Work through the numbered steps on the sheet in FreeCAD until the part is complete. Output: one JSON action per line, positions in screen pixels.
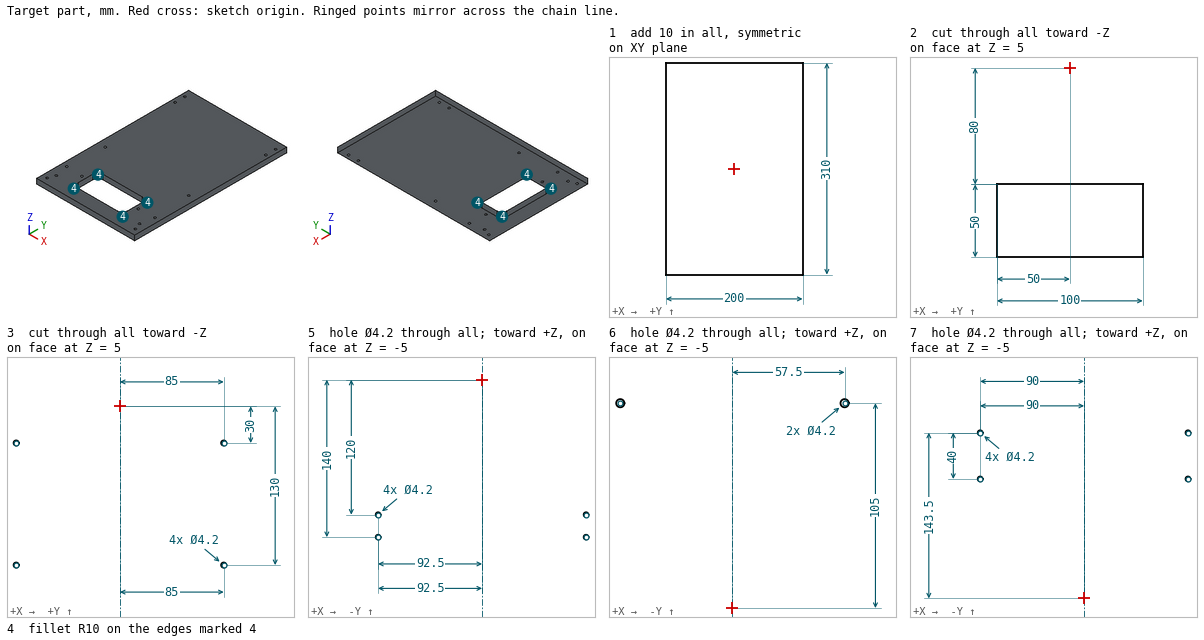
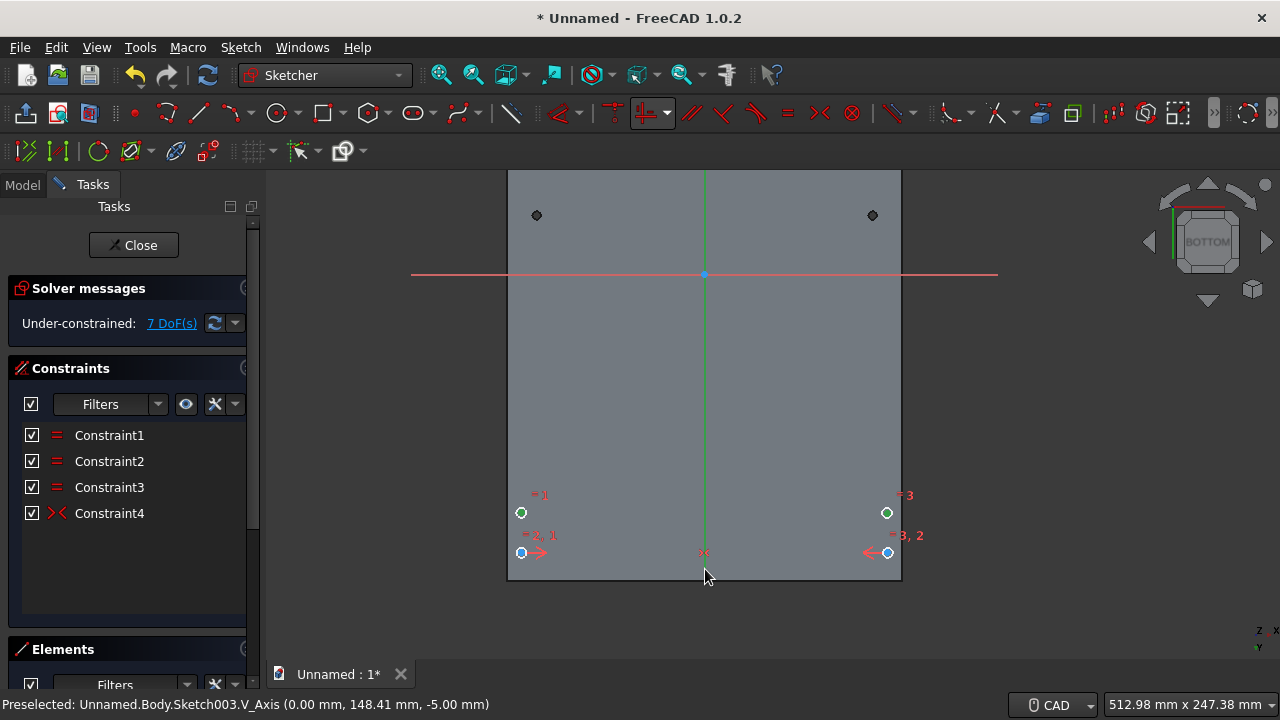
{"action": "left_click", "coordinate": [820, 114]}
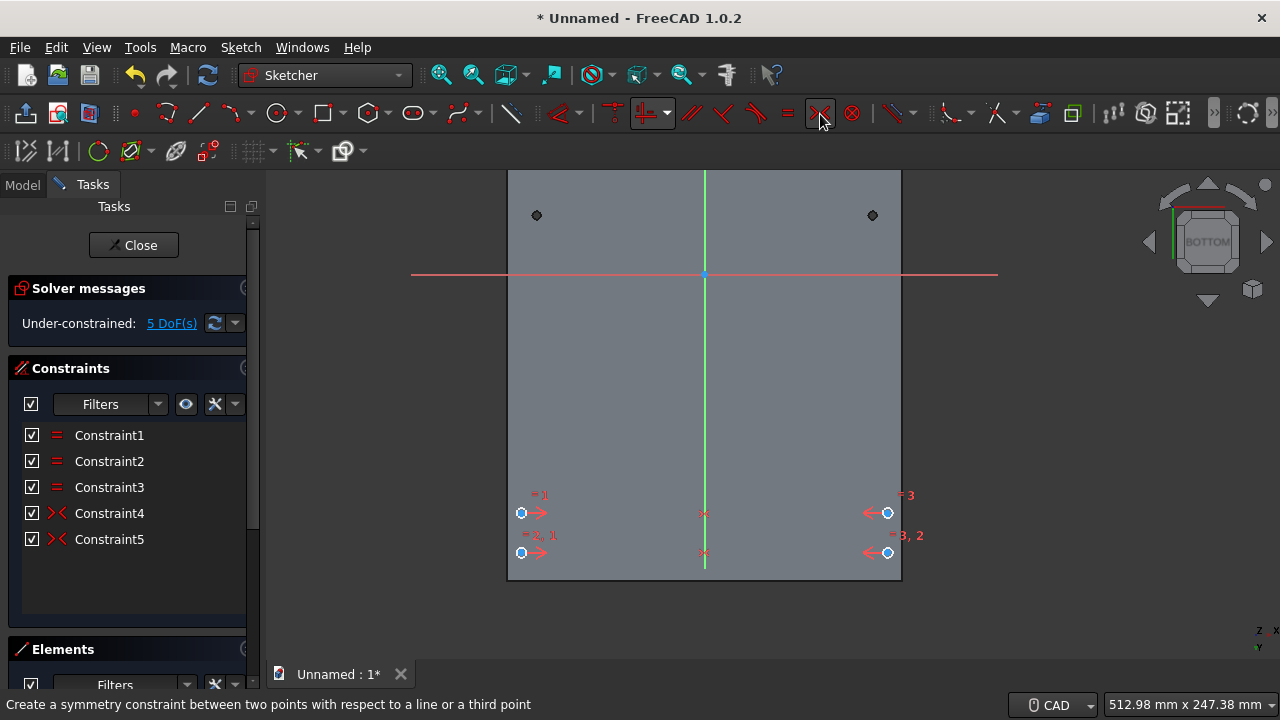
{"action": "left_click", "coordinate": [558, 114]}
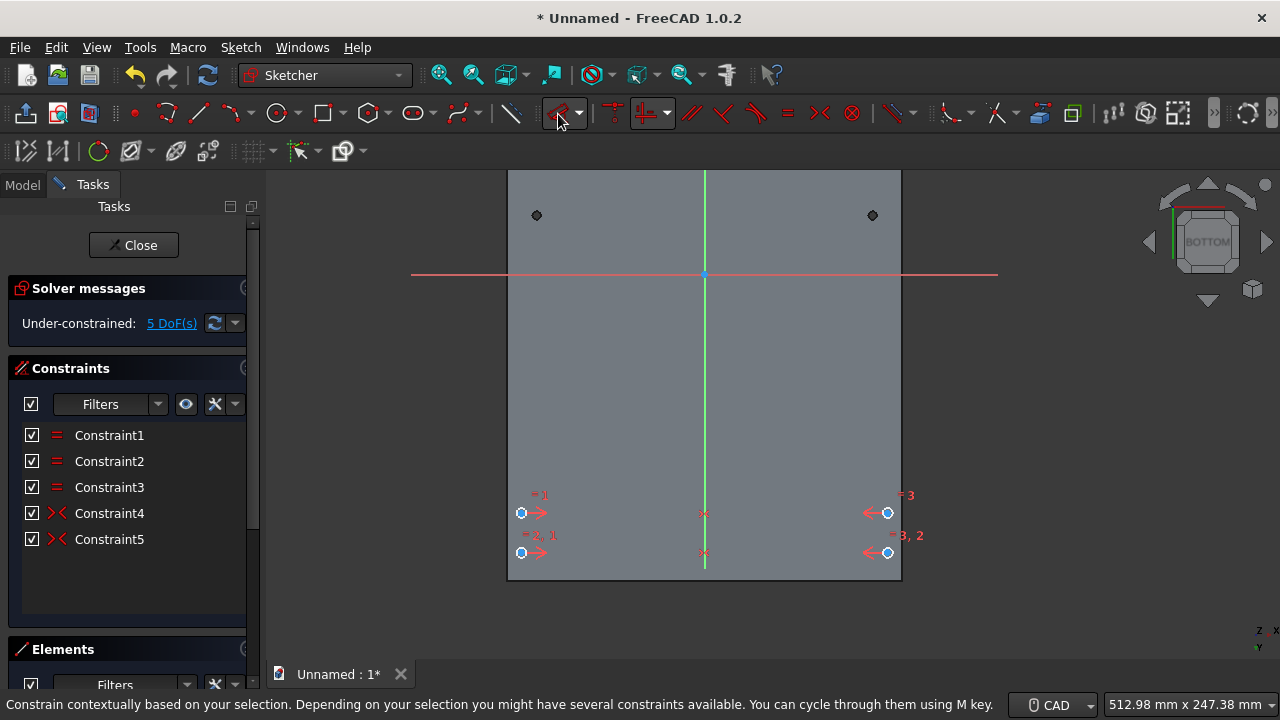
{"action": "scroll", "coordinate": [525, 510], "scroll_direction": "up", "scroll_amount": 8}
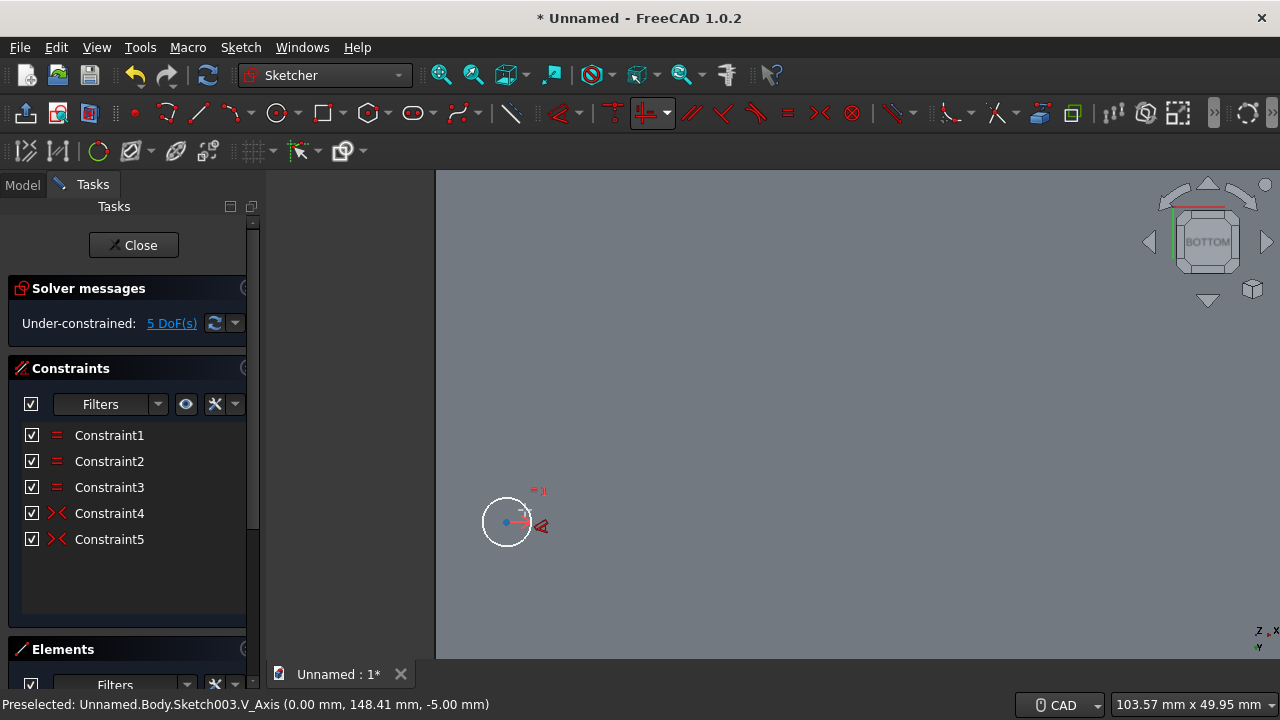
{"action": "left_click", "coordinate": [524, 505]}
{"action": "left_click", "coordinate": [547, 482]}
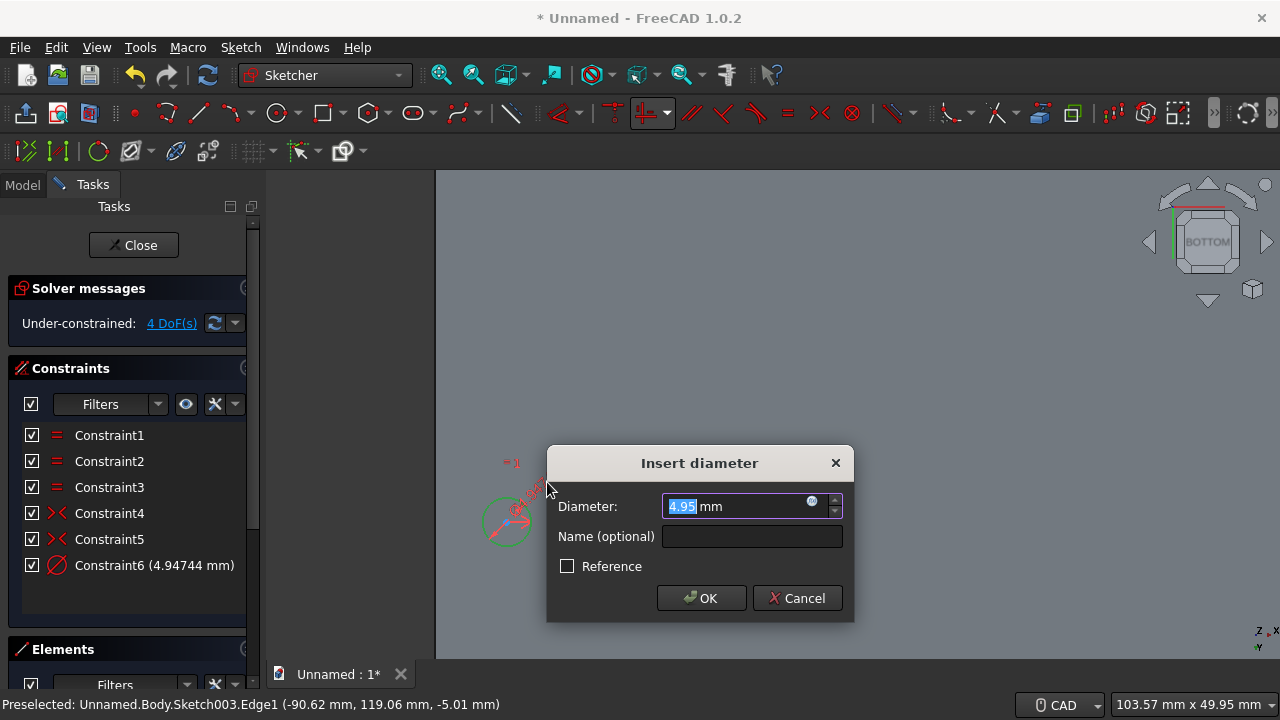
{"action": "type", "text": "4.2"}
{"action": "key", "text": "Return"}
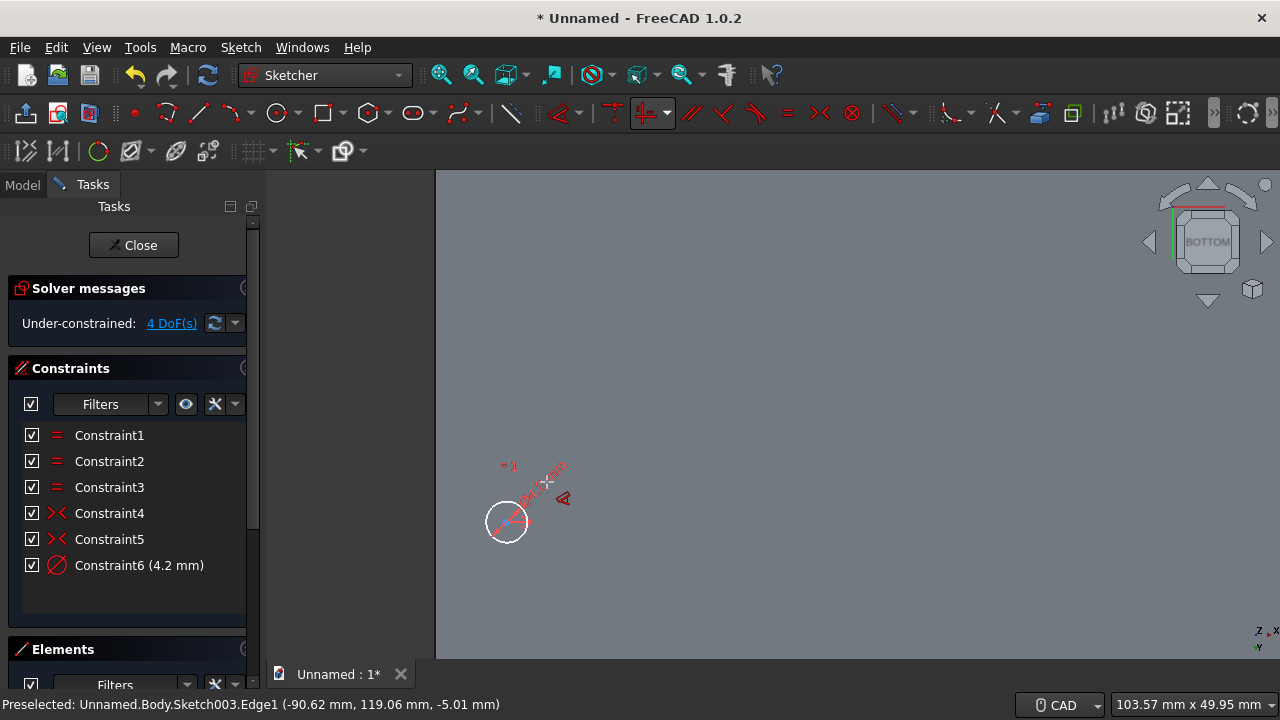
{"action": "scroll", "coordinate": [525, 510], "scroll_direction": "down", "scroll_amount": 8}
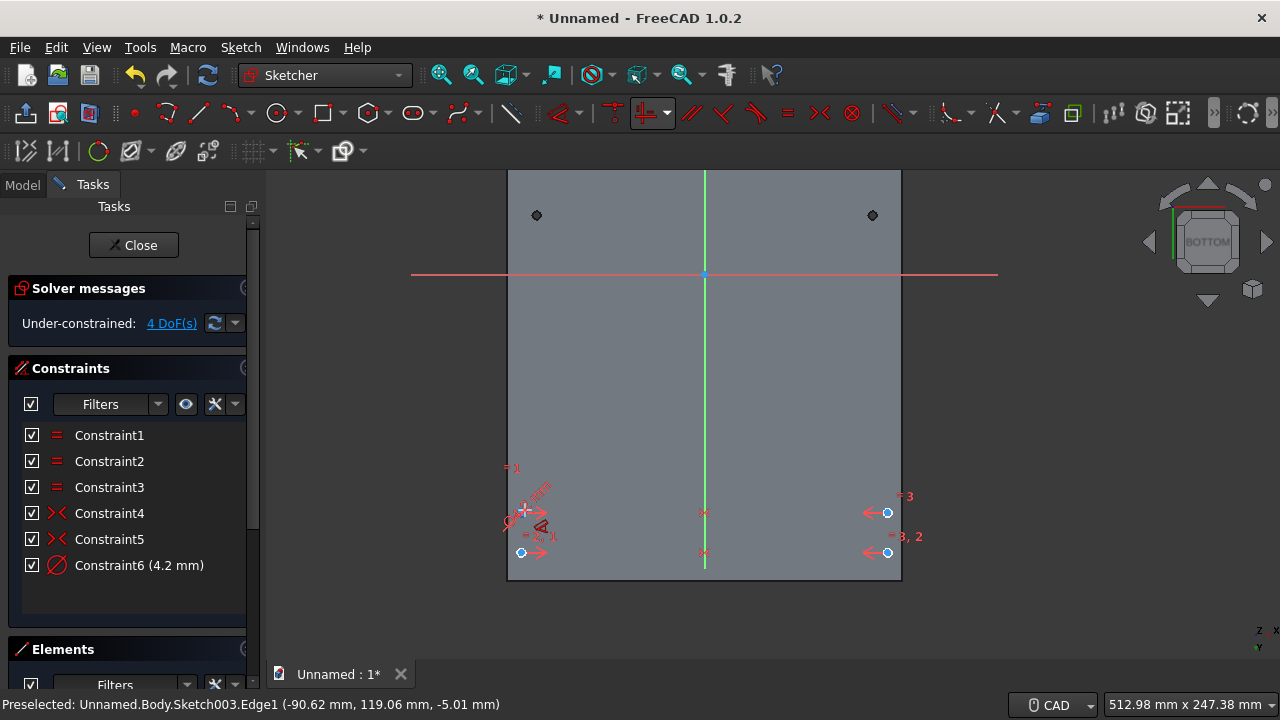
{"action": "left_click", "coordinate": [522, 513]}
{"action": "left_click", "coordinate": [488, 394]}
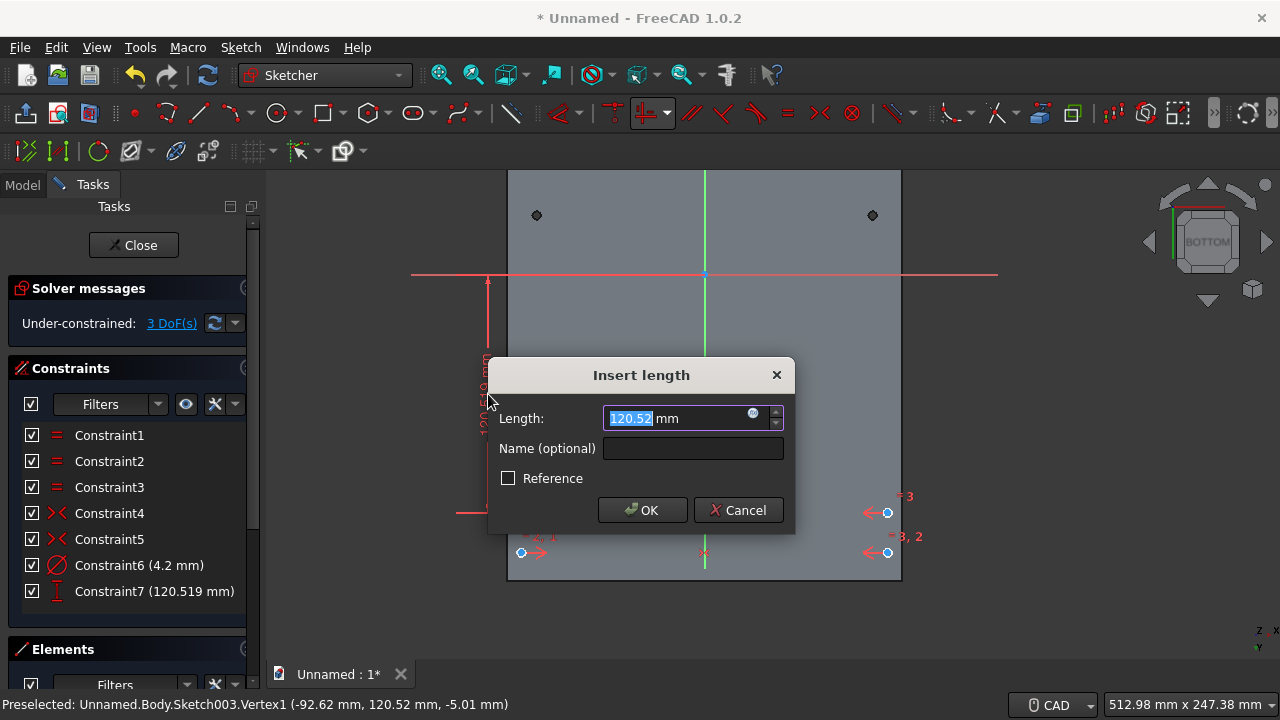
{"action": "type", "text": "120"}
{"action": "key", "text": "Return"}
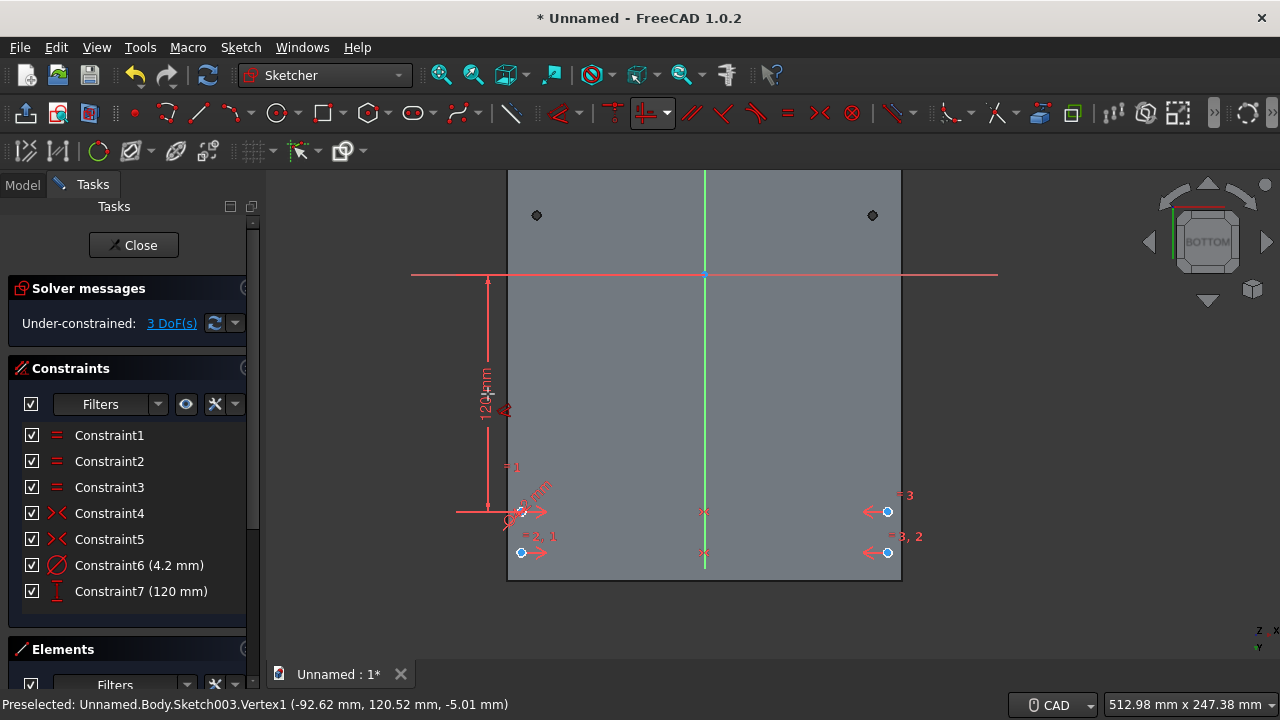
{"action": "left_click", "coordinate": [521, 553]}
{"action": "left_click", "coordinate": [487, 350]}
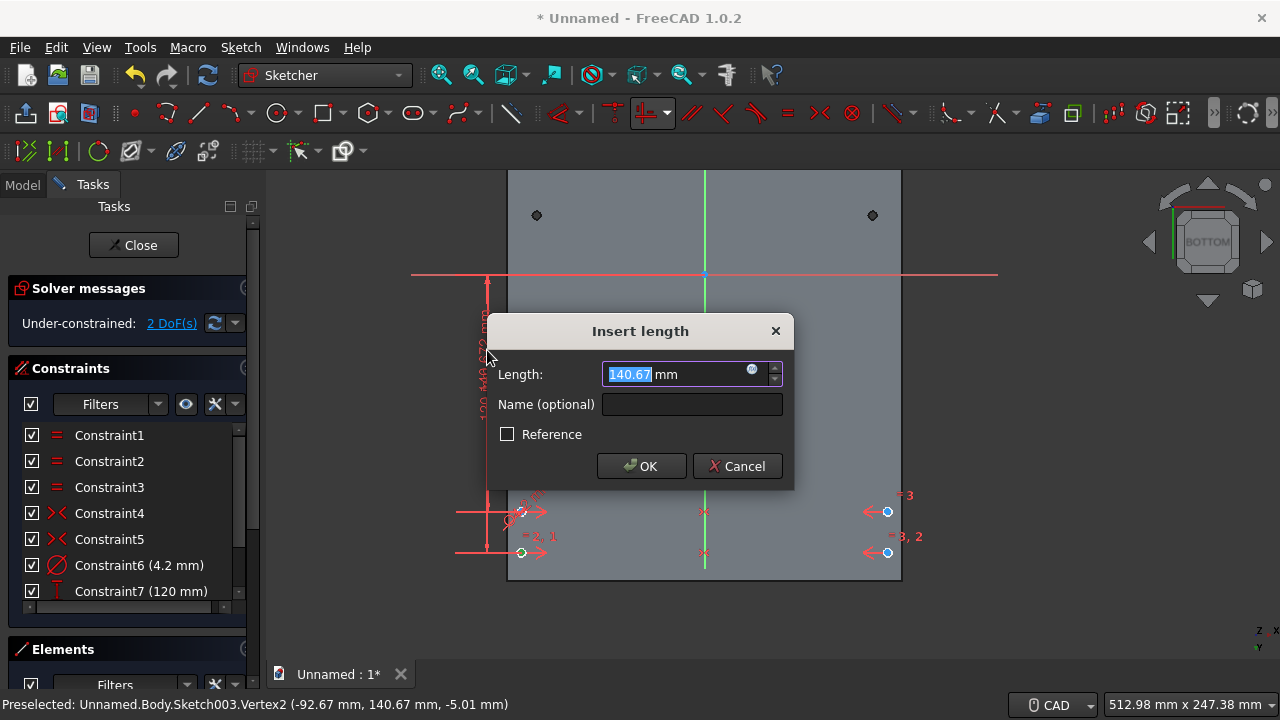
{"action": "type", "text": "140"}
{"action": "key", "text": "Return"}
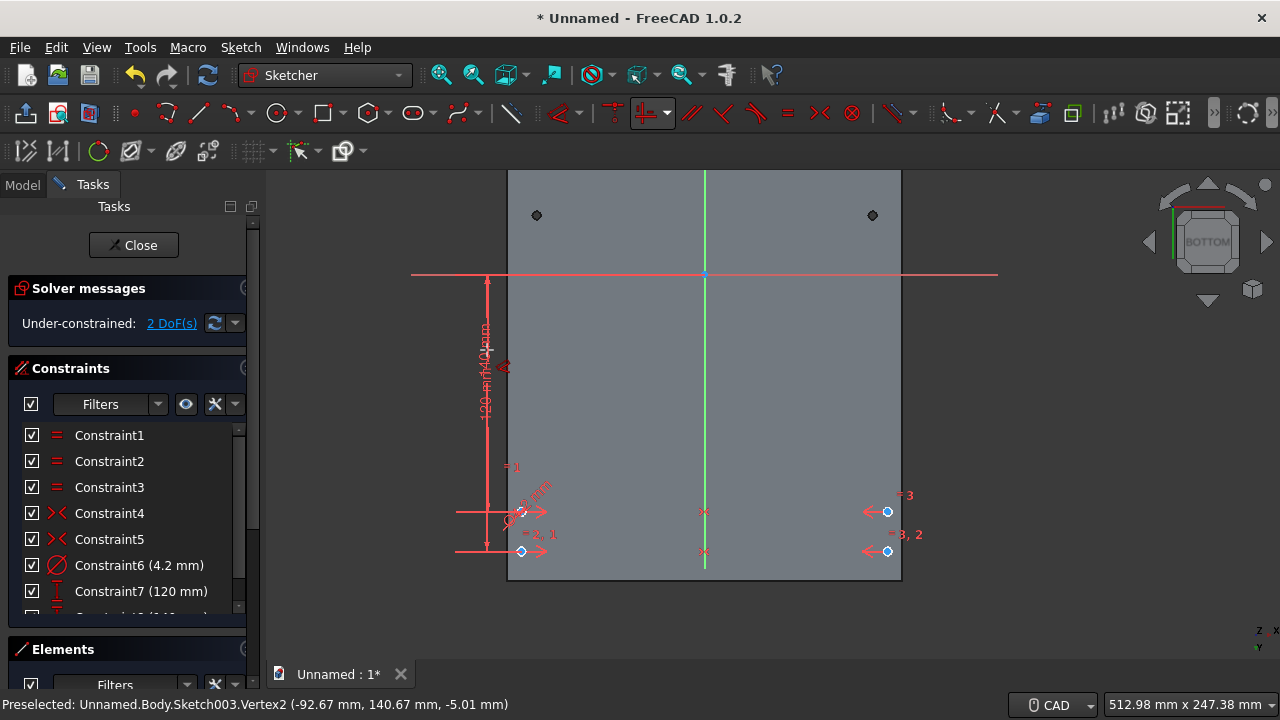
{"action": "left_click", "coordinate": [522, 512]}
{"action": "left_click", "coordinate": [613, 241]}